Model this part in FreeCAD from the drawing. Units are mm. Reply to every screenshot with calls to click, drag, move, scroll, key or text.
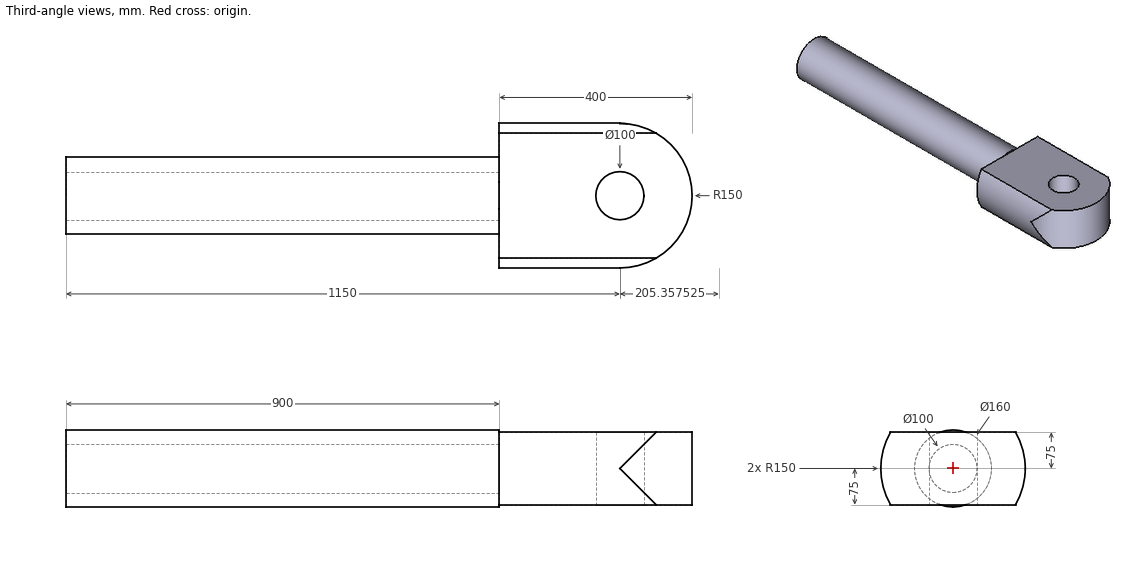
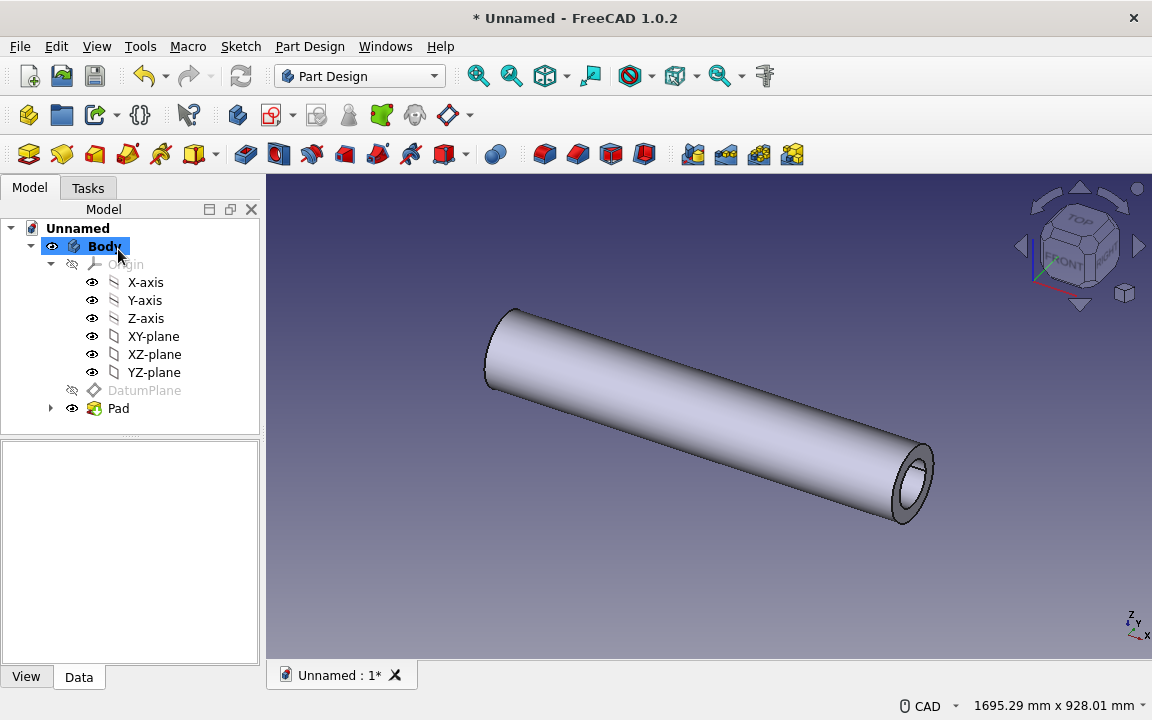
key(0)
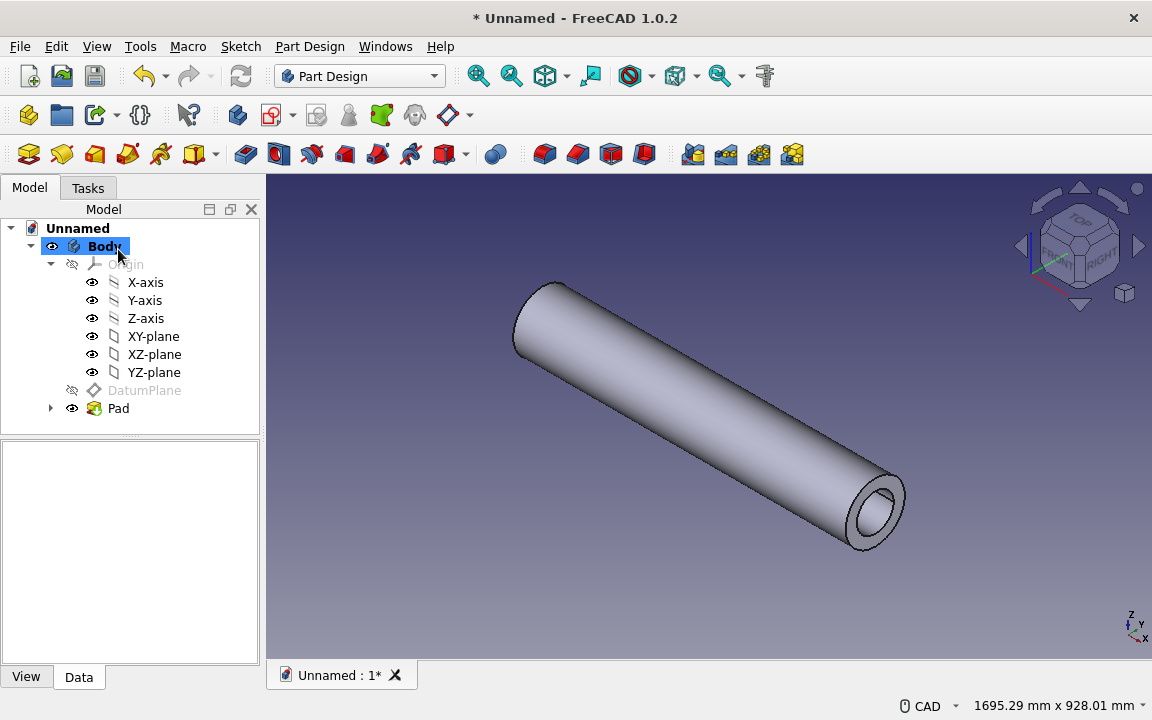
key(3)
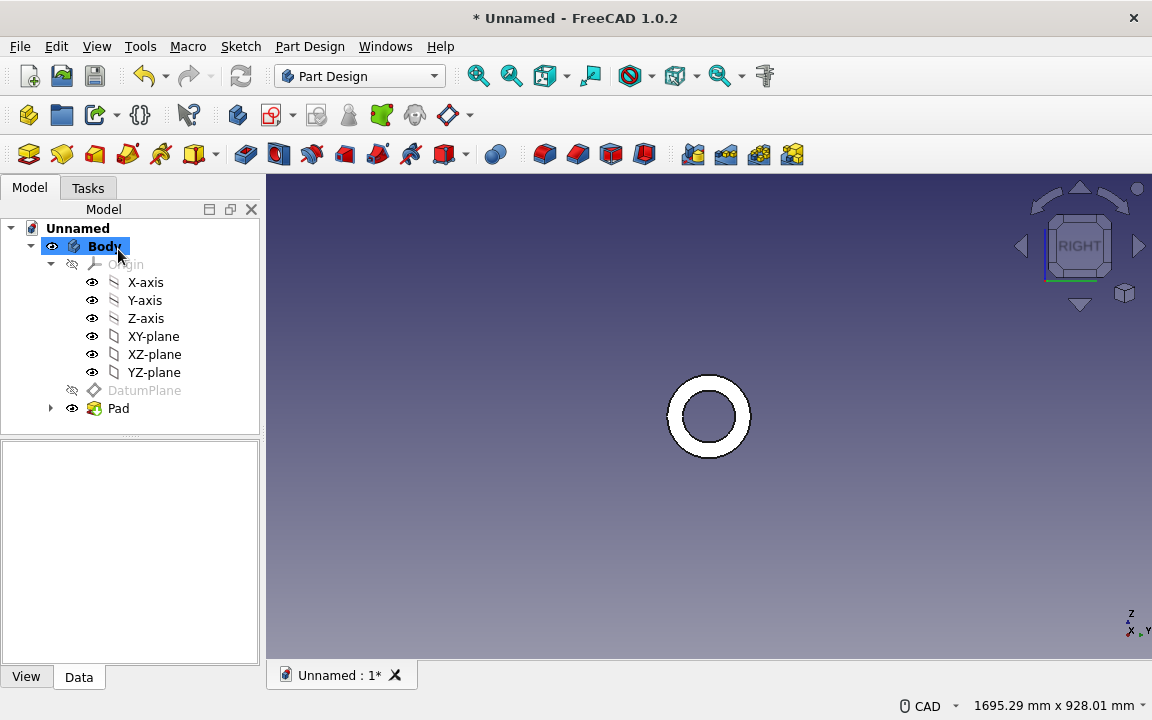
key(v)
key(f)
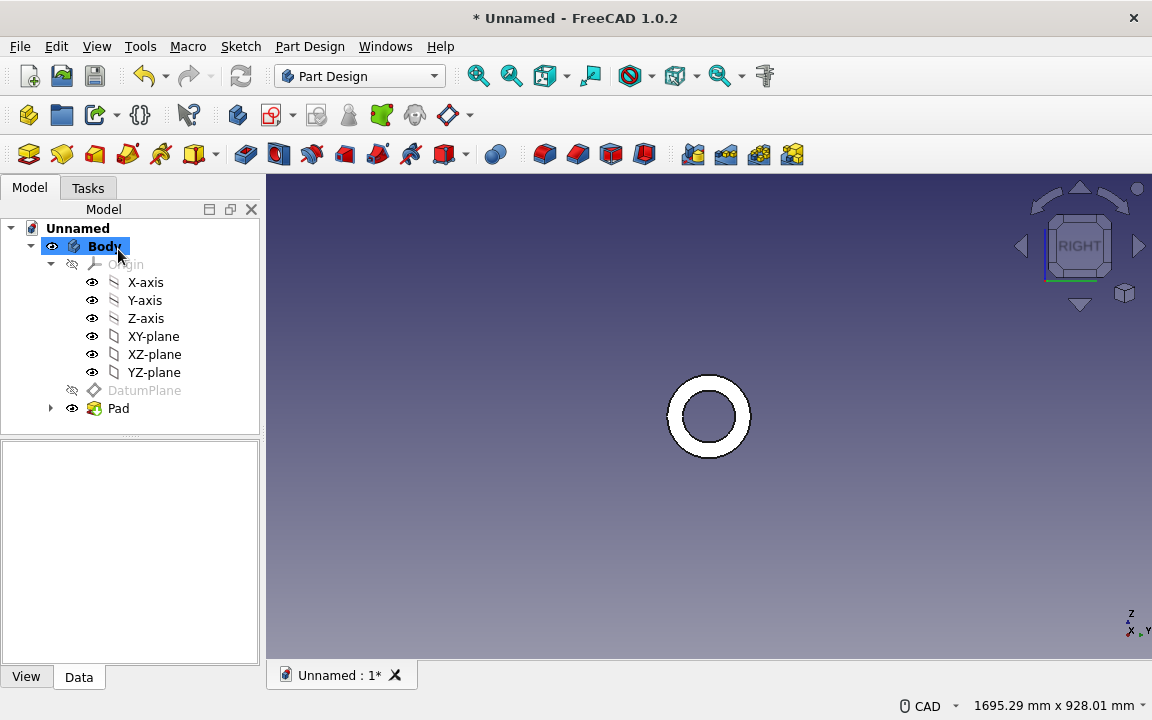
key(1)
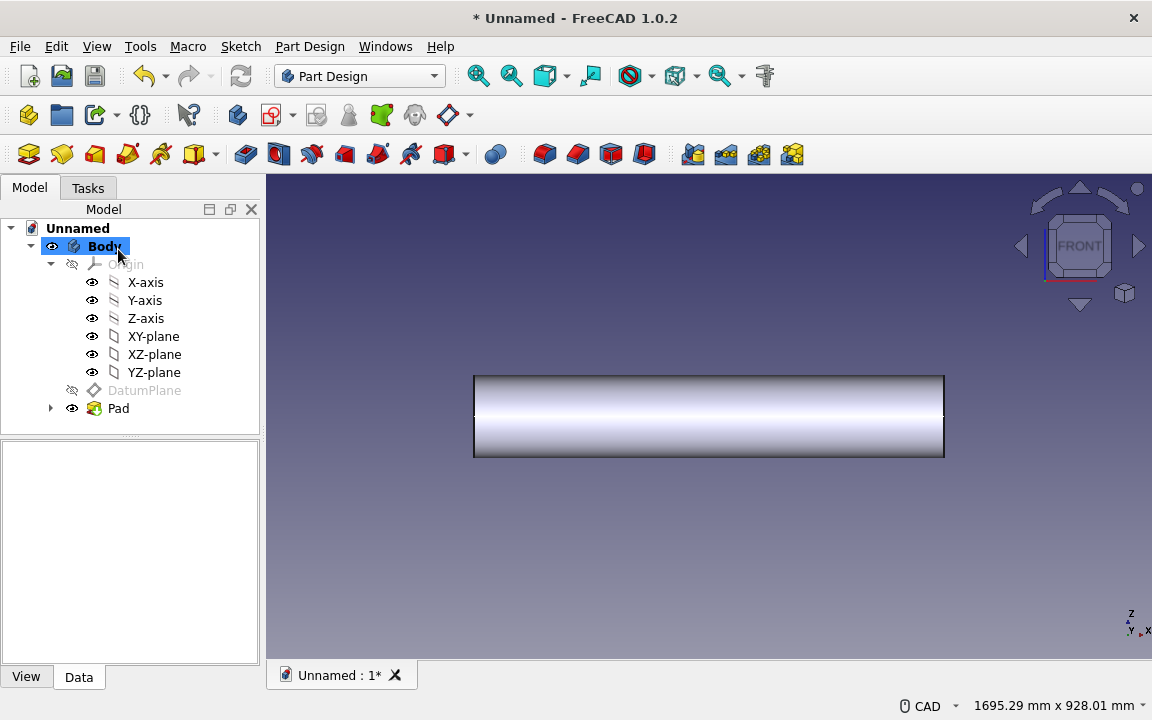
click(137, 372)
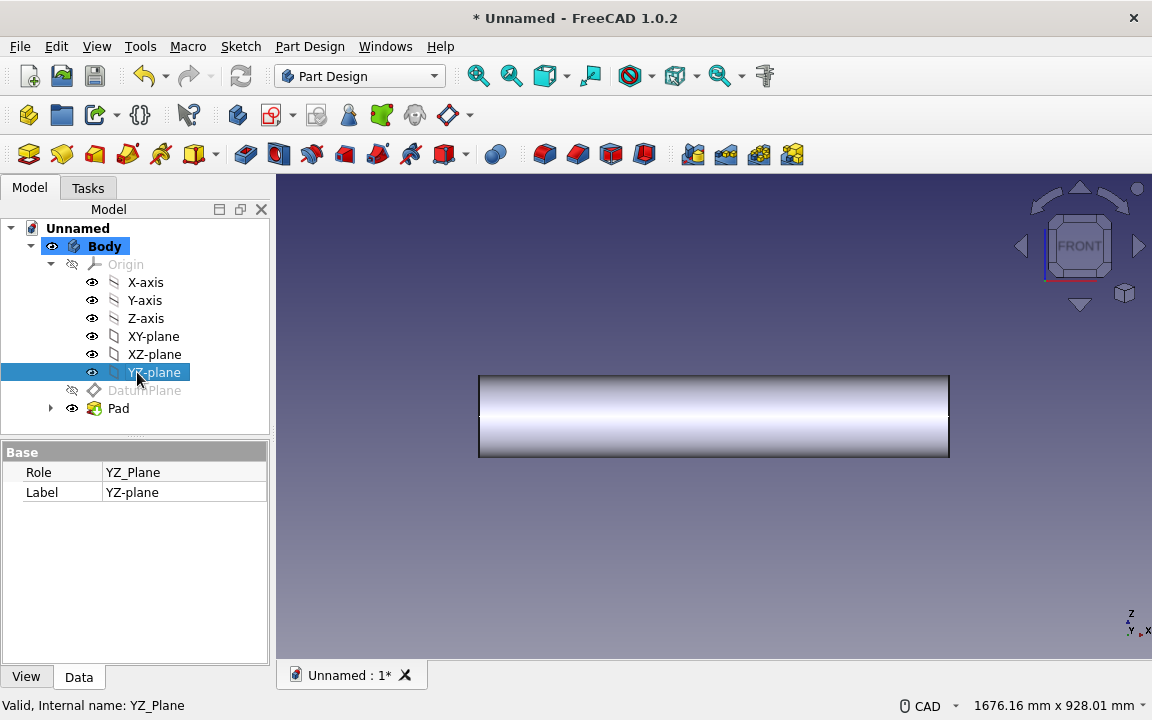
click(448, 116)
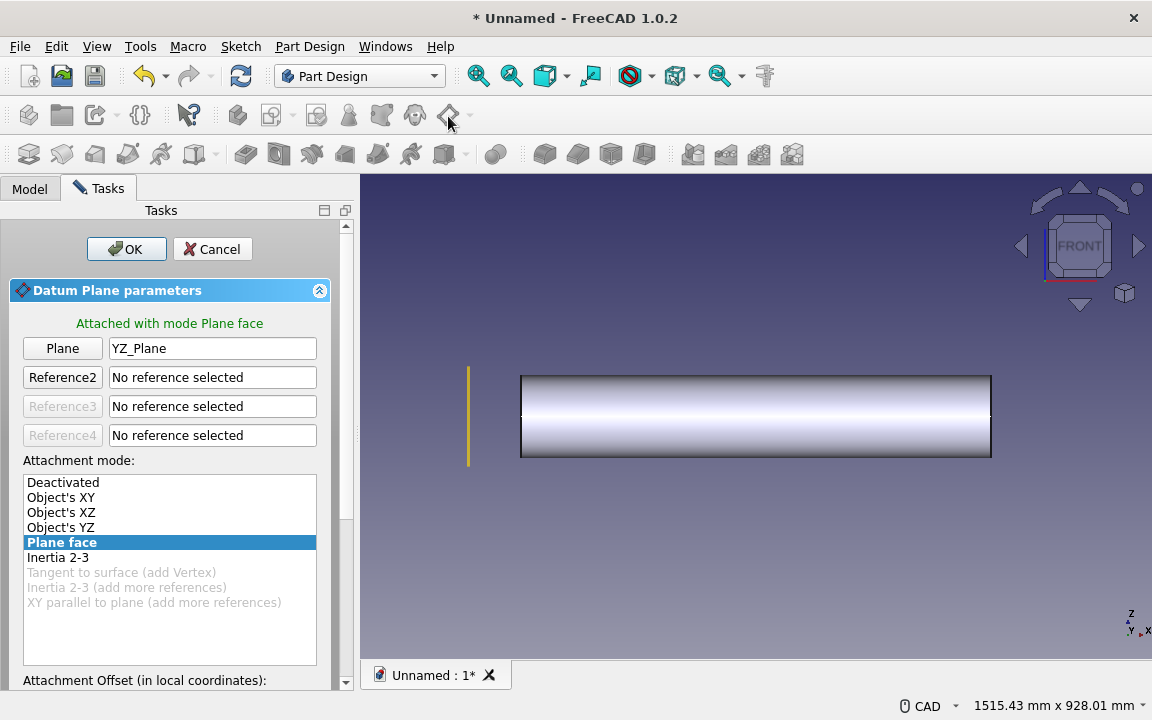
scroll(346, 455, down, 3)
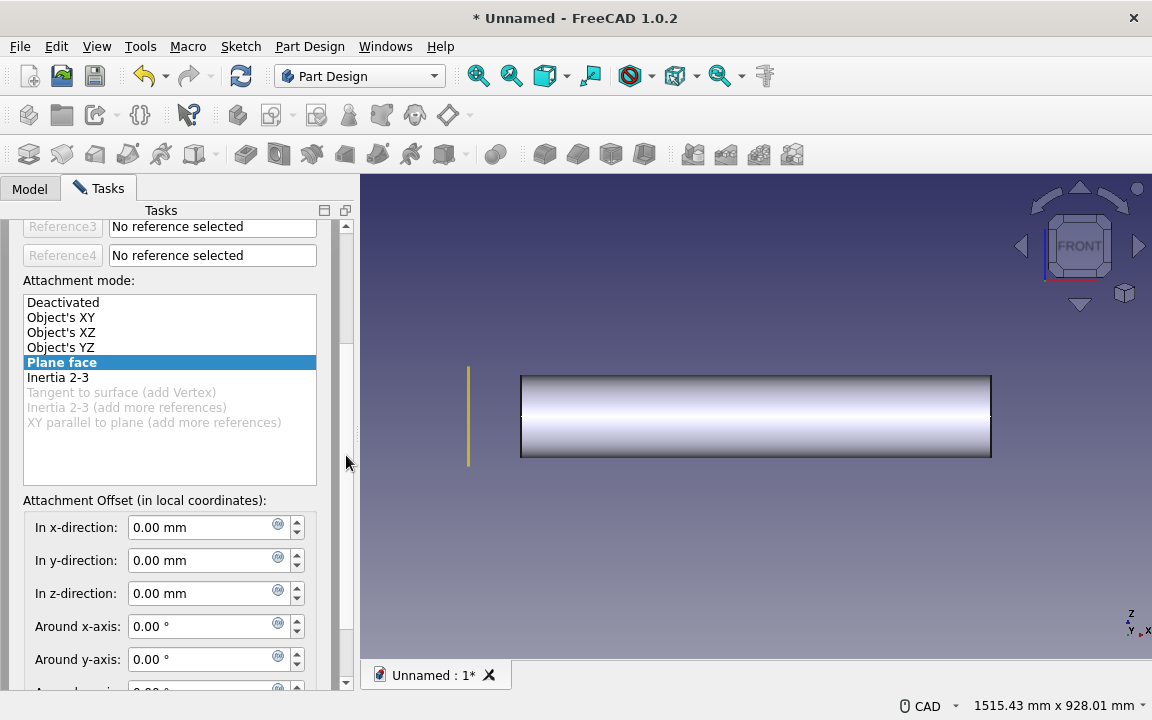
triple_click(210, 594)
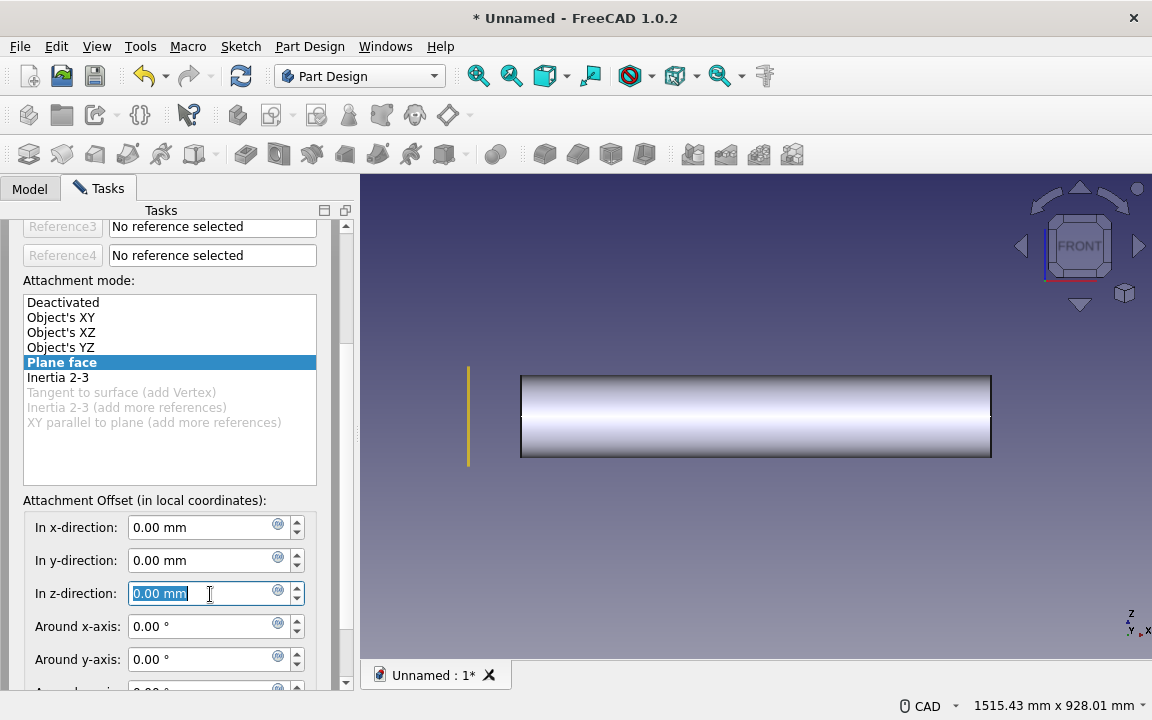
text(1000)
key(Tab)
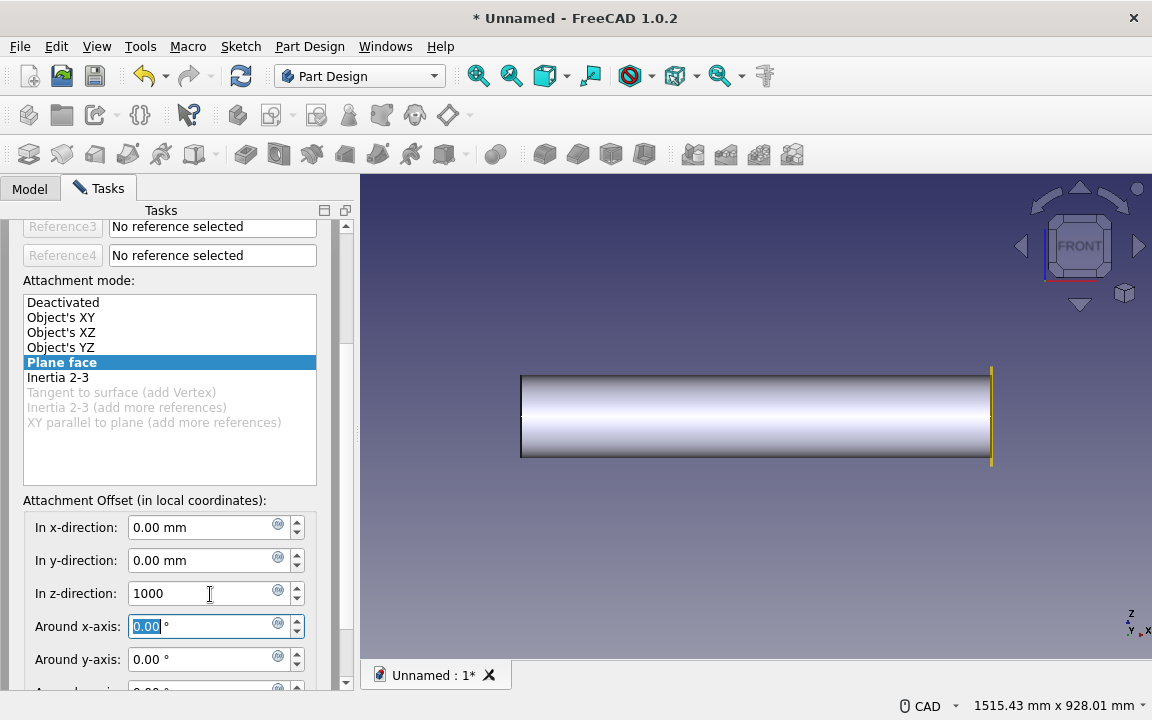
scroll(346, 455, up, 4)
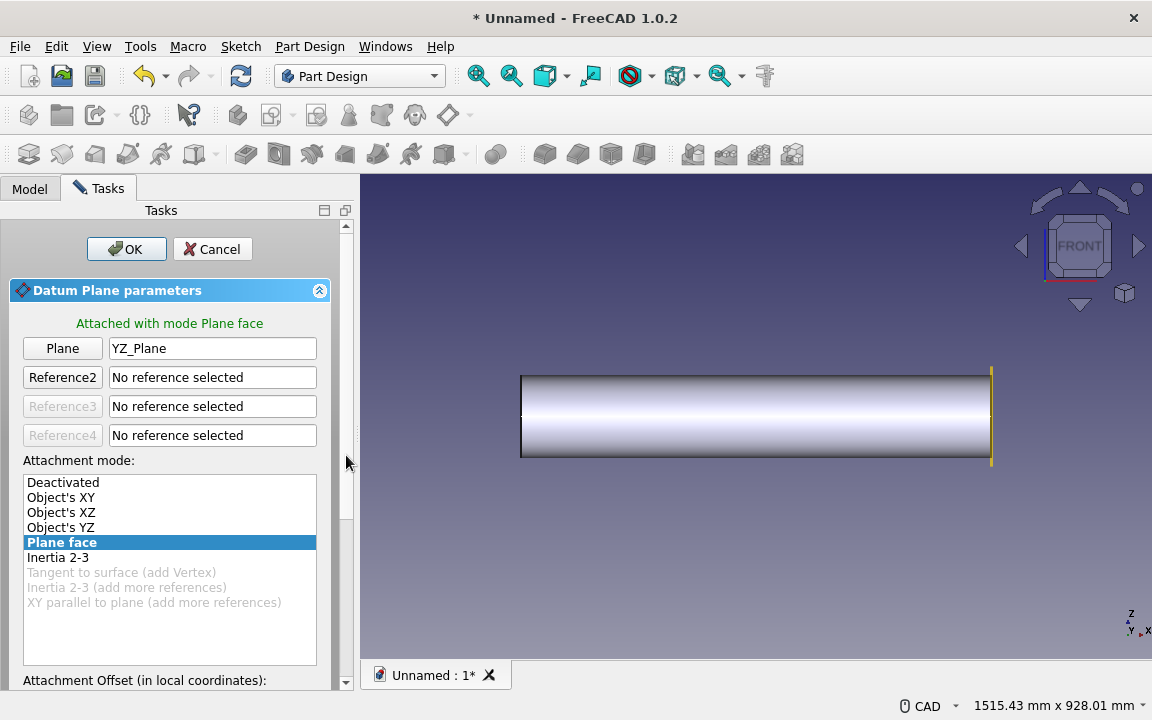
click(127, 249)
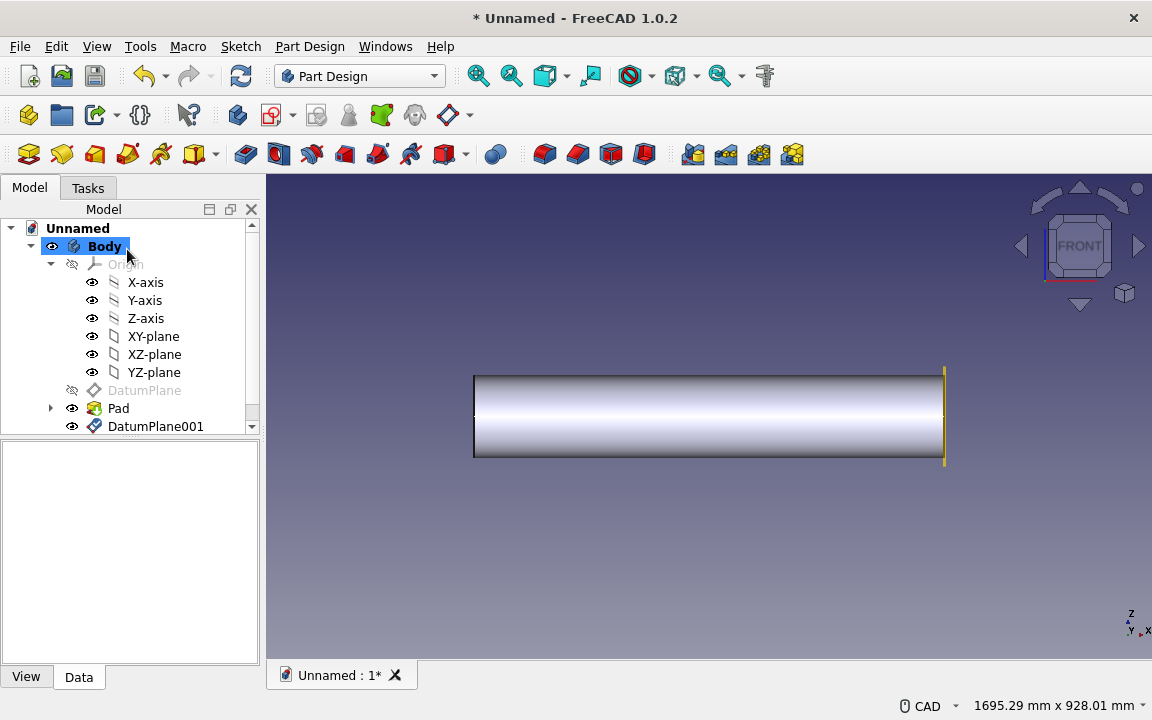
click(117, 426)